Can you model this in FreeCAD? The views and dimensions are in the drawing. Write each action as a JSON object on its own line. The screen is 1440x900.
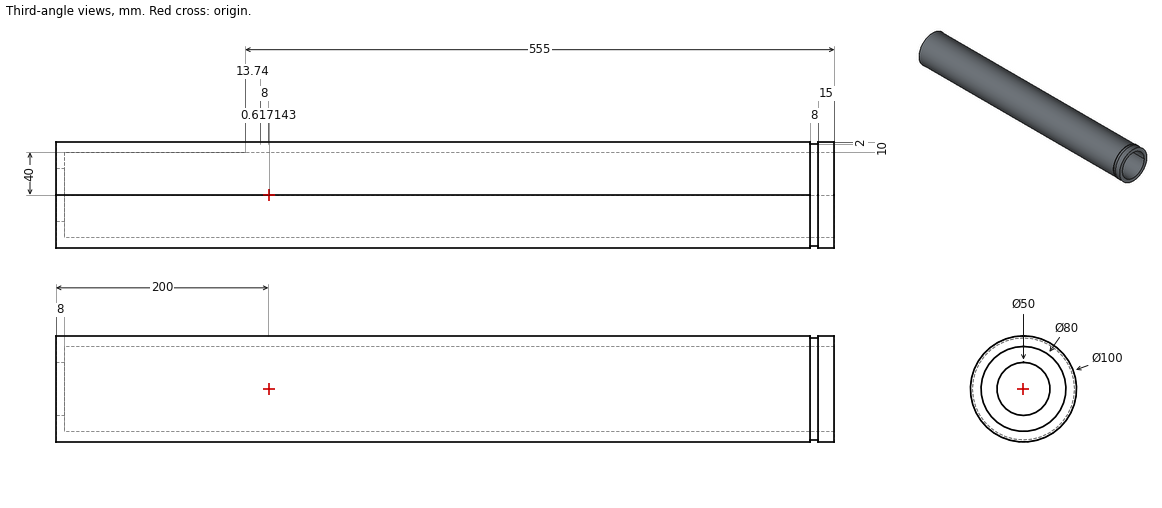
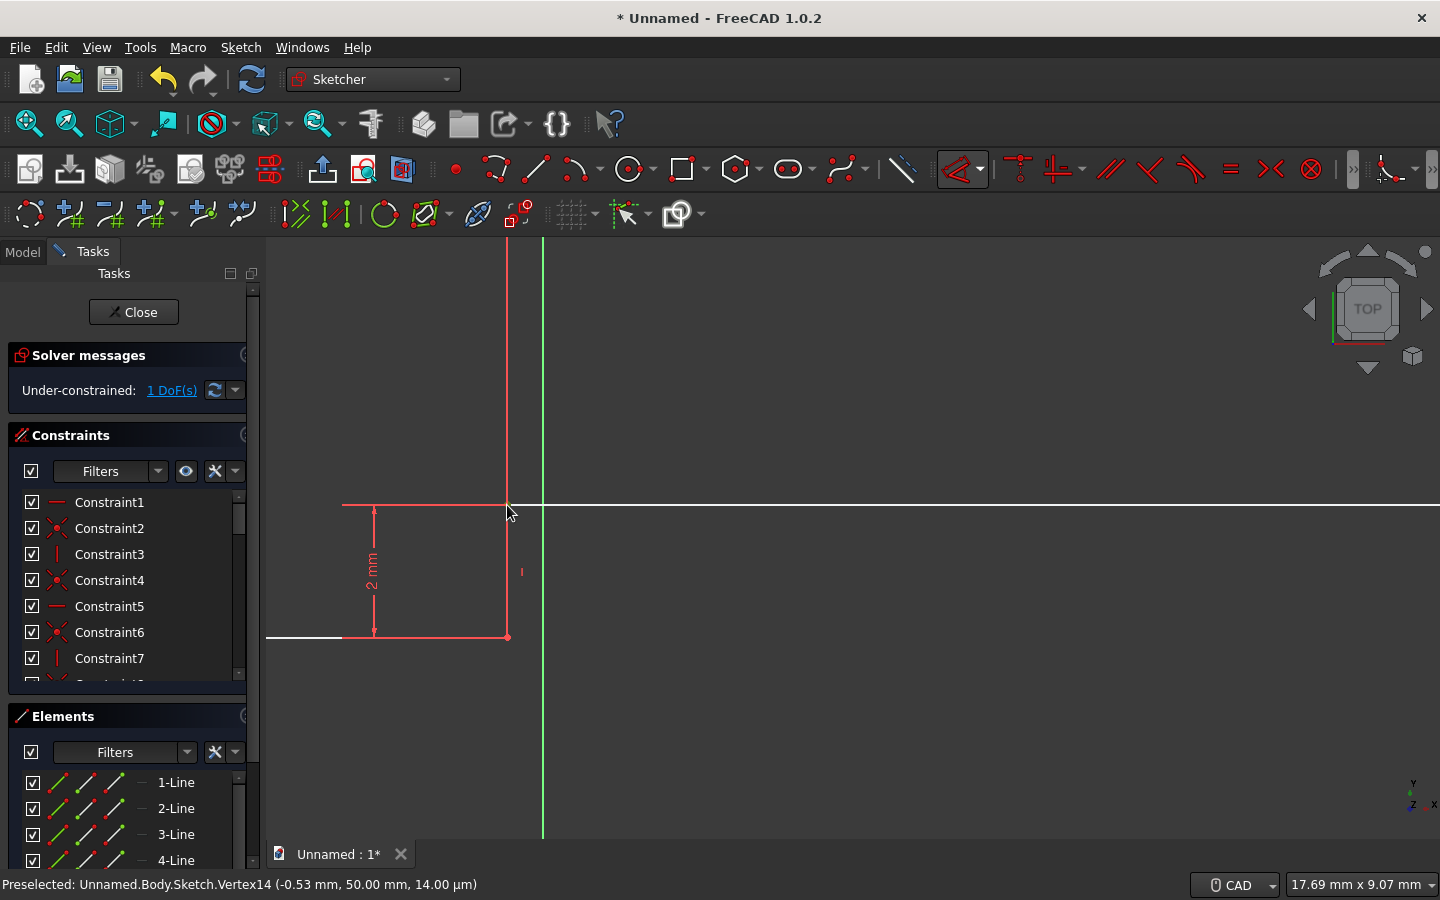
{"action": "left_click", "coordinate": [982, 170]}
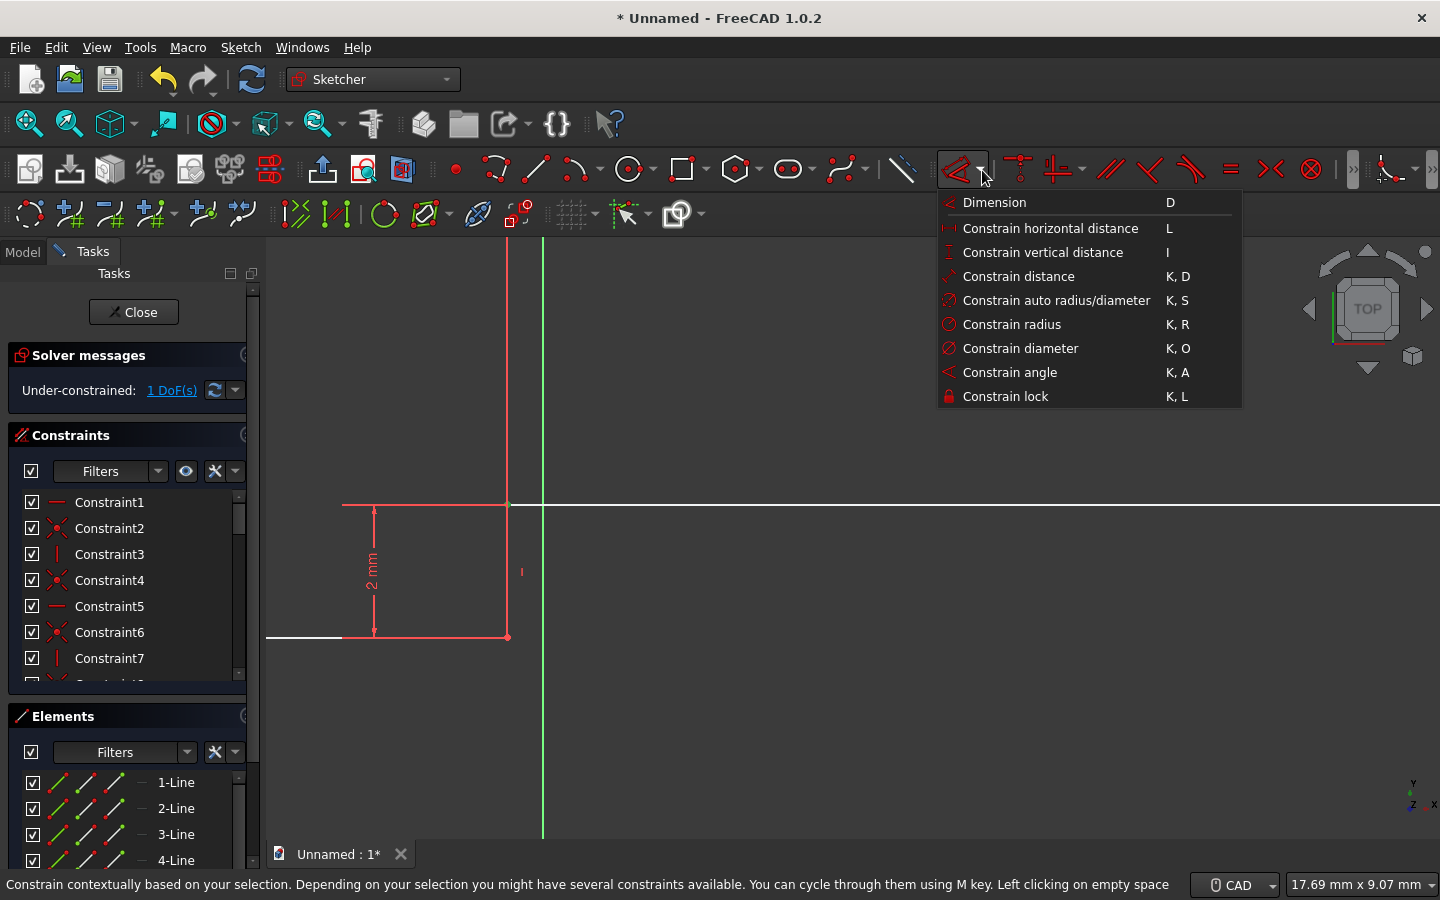
{"action": "left_click", "coordinate": [1090, 228]}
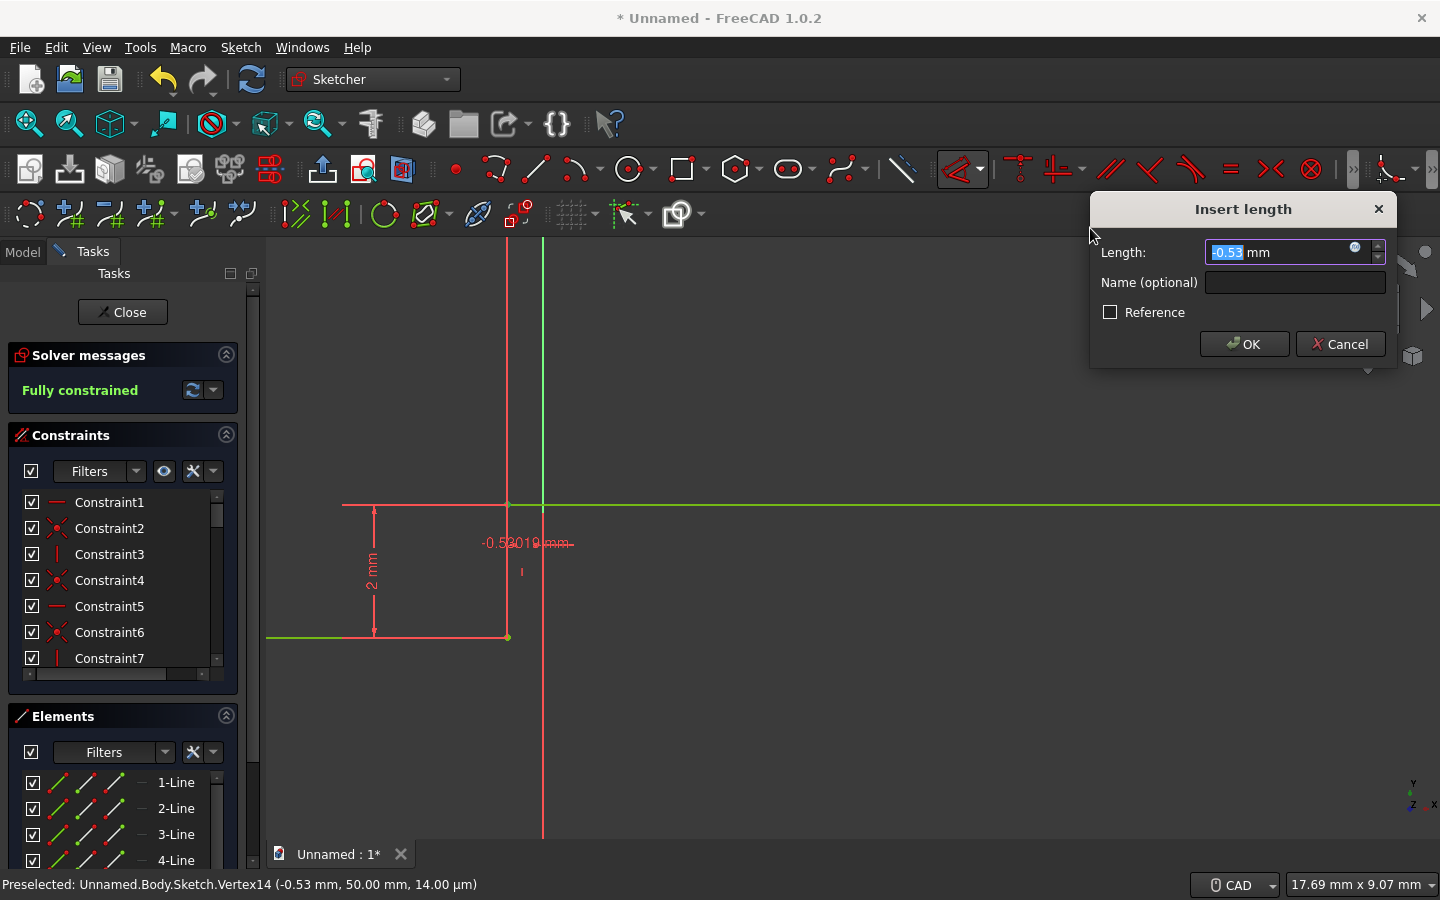
{"action": "type", "text": "-0.617143"}
{"action": "key", "text": "Return"}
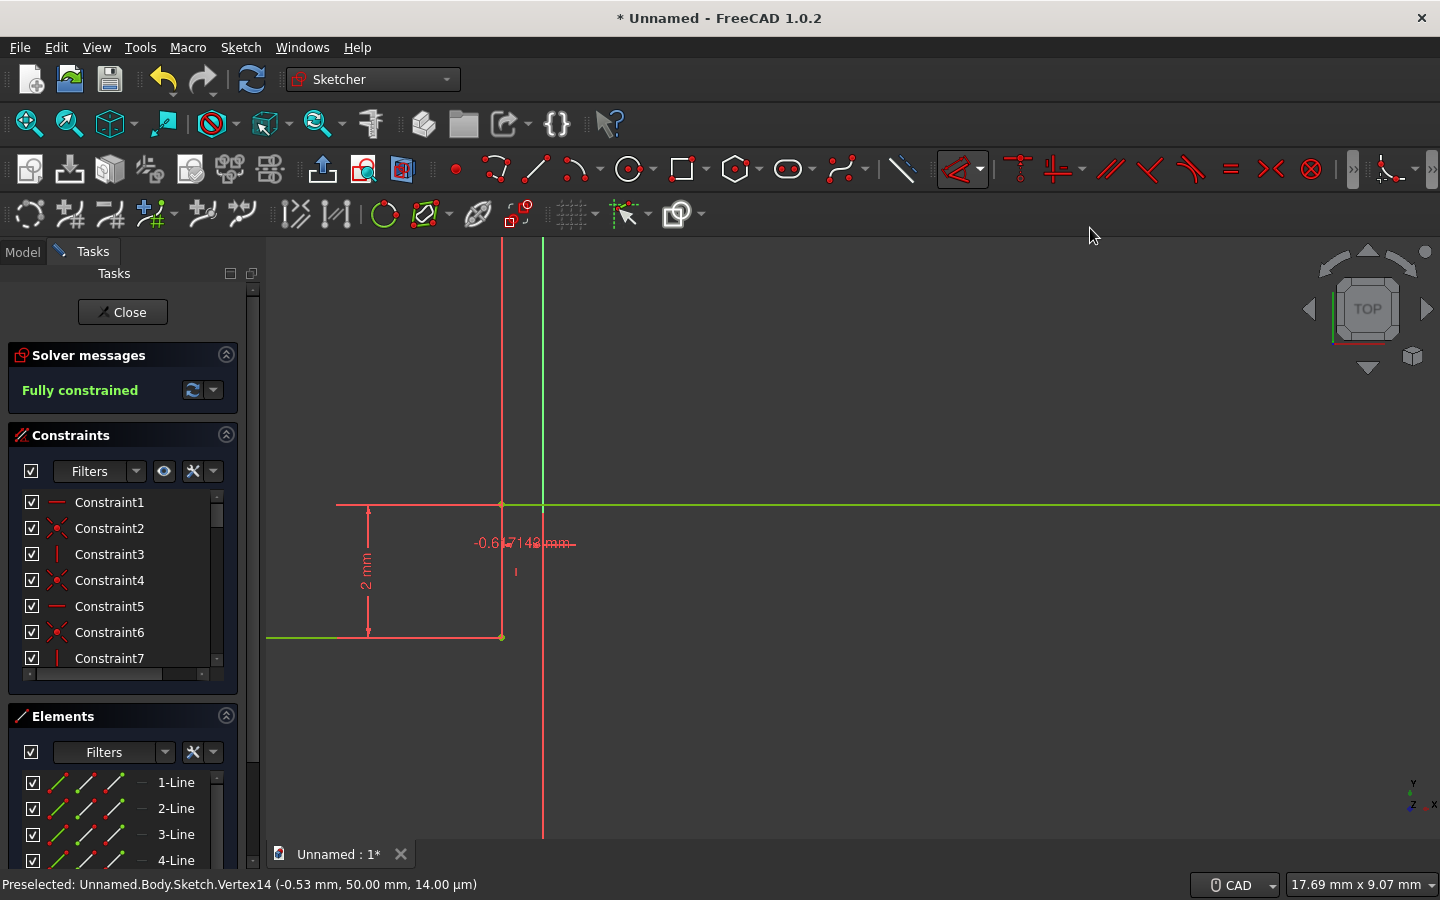
{"action": "left_click", "coordinate": [123, 312]}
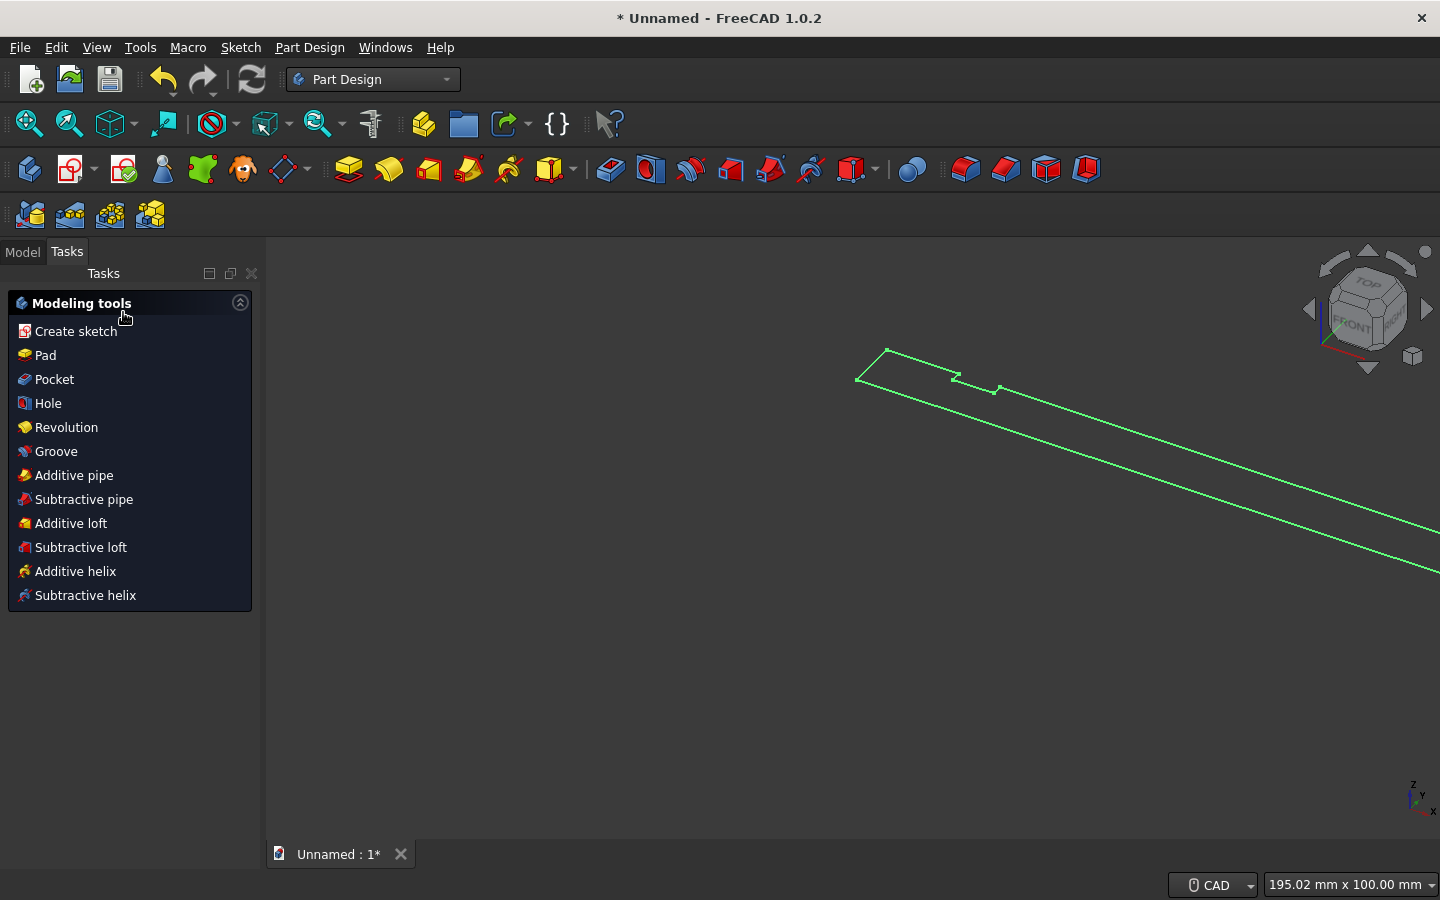
{"action": "left_click", "coordinate": [390, 170]}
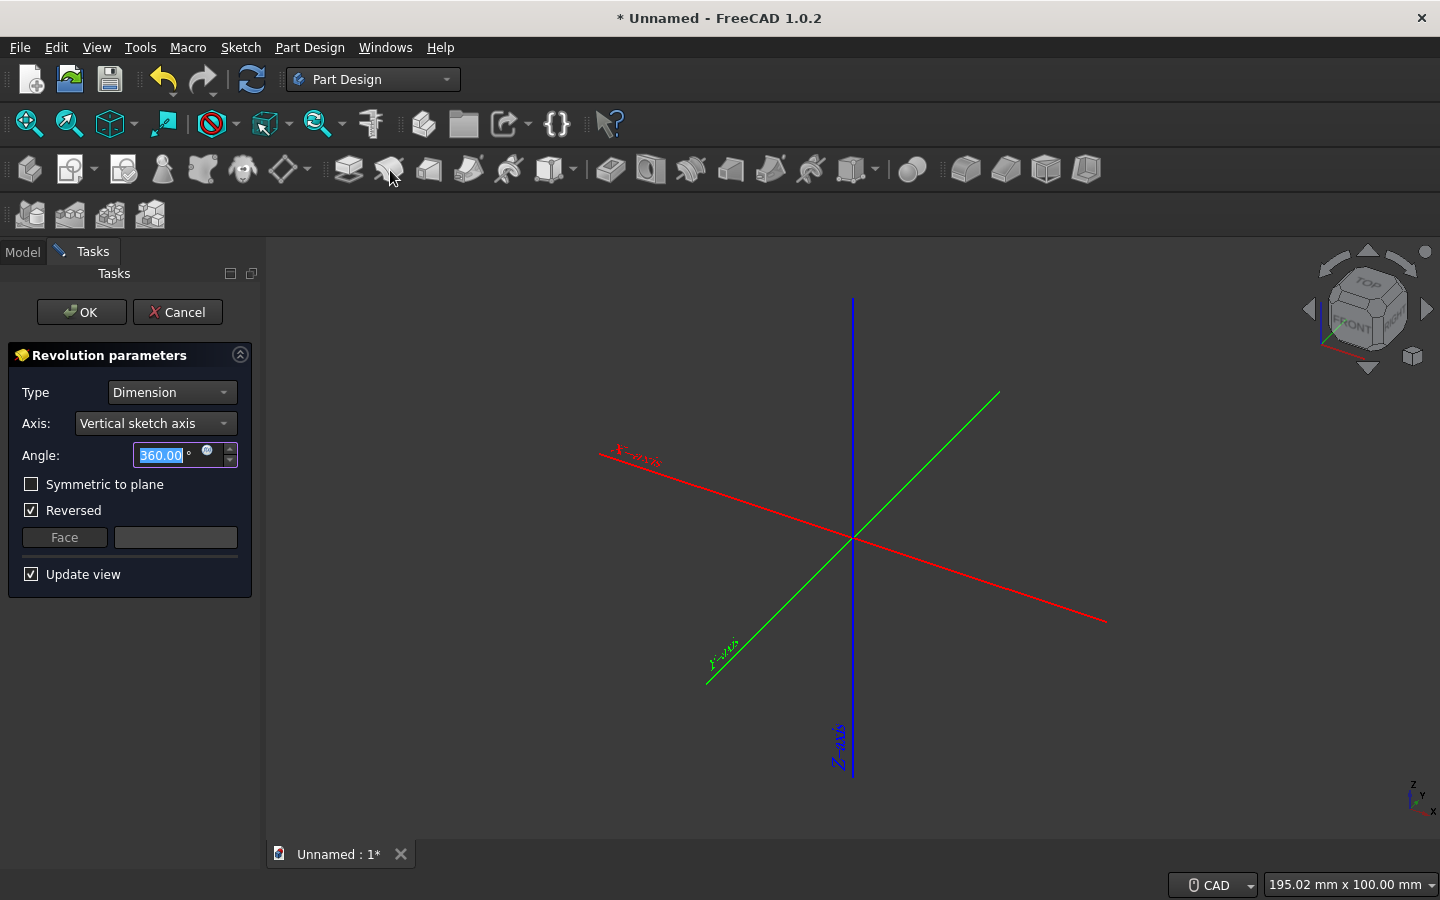
{"action": "left_click", "coordinate": [156, 424]}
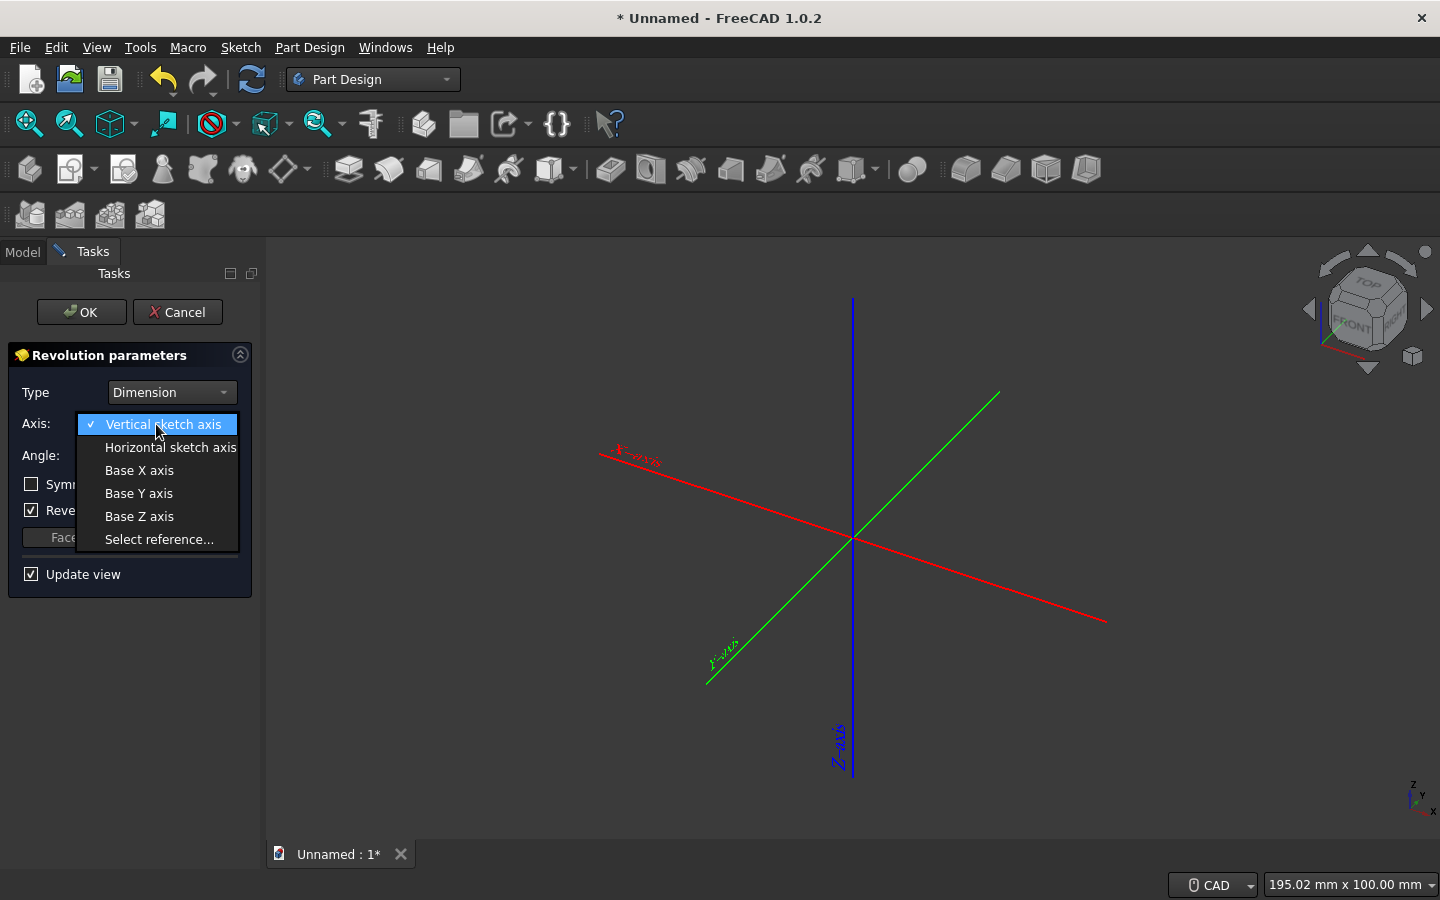
{"action": "left_click", "coordinate": [156, 448]}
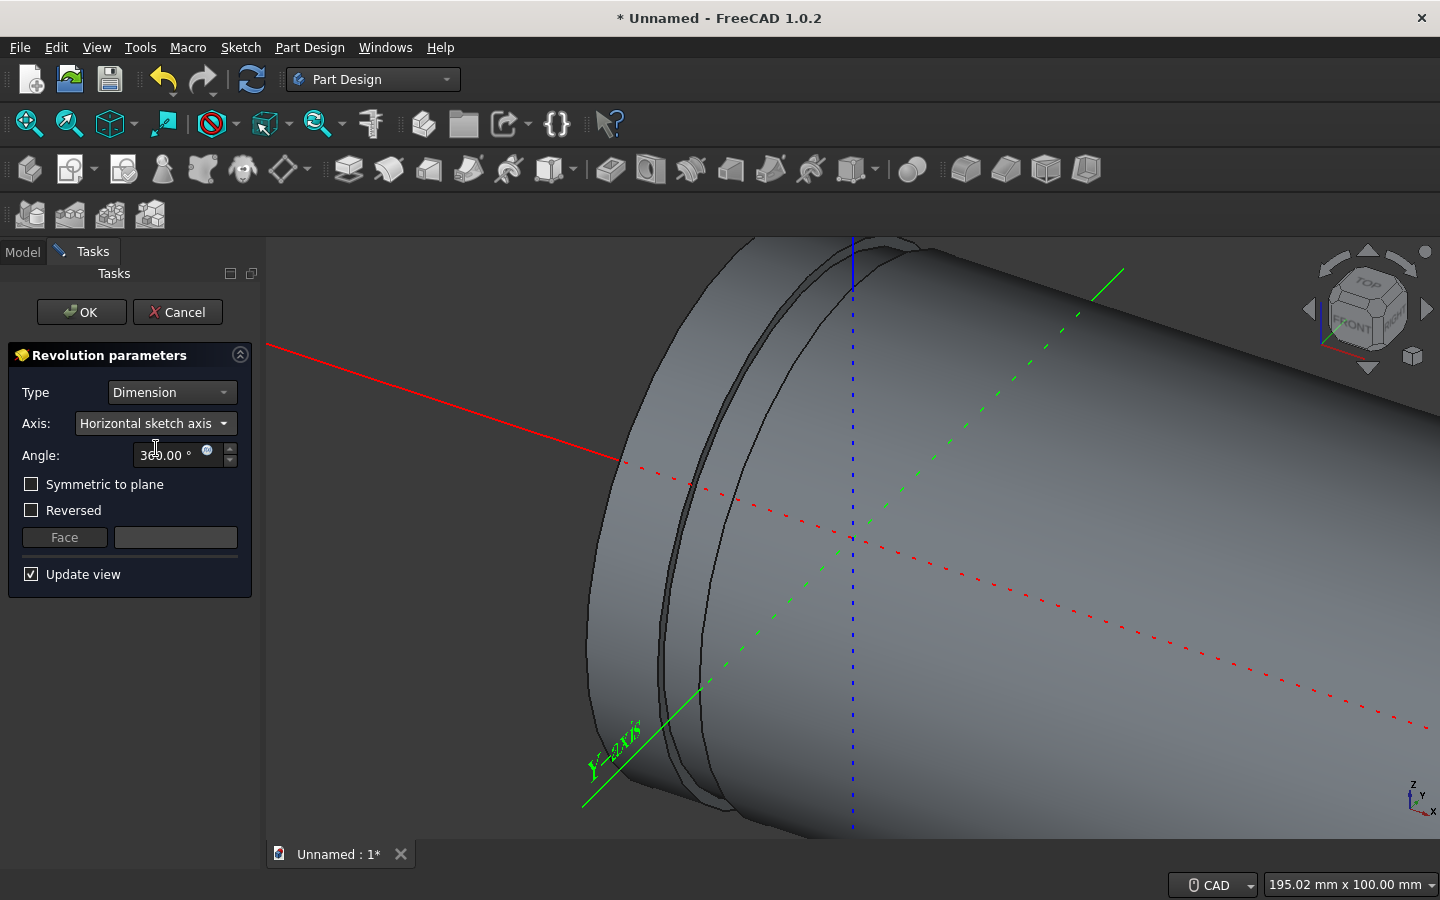
{"action": "left_click", "coordinate": [82, 312]}